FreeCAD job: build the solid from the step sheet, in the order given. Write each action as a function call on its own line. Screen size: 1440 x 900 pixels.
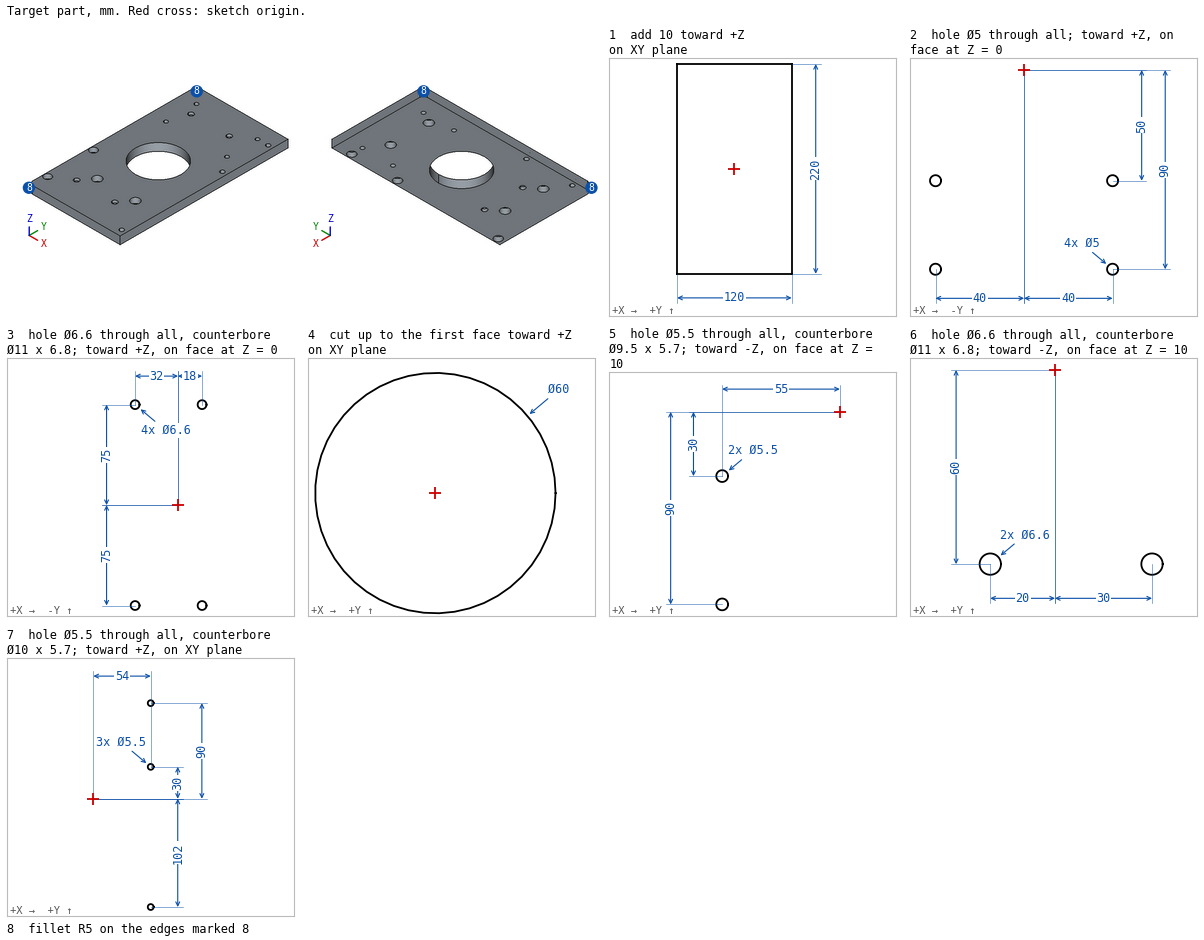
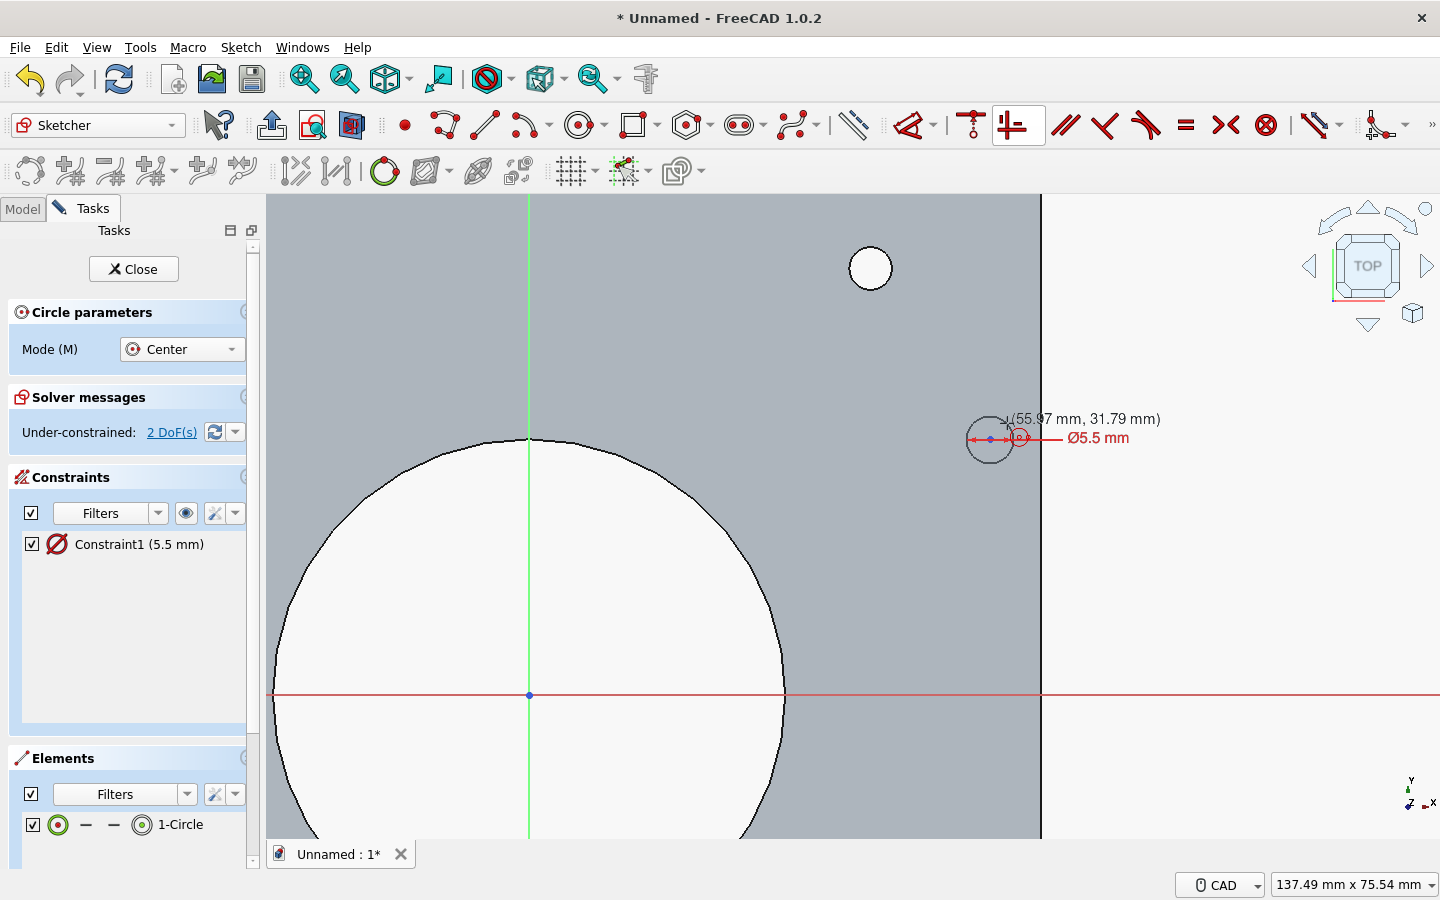
scroll(789, 441, down, 7)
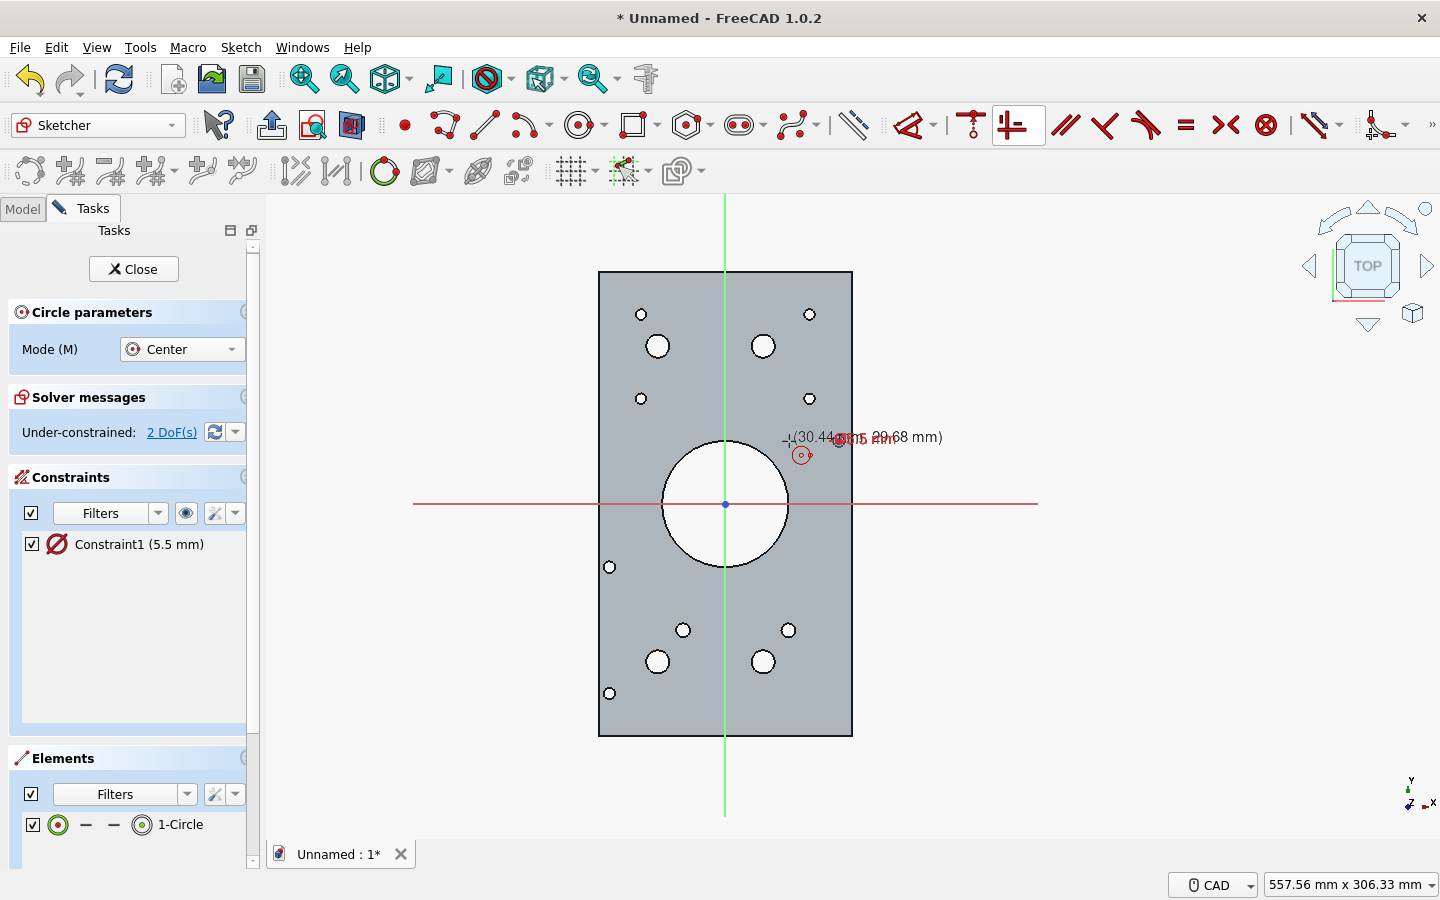
scroll(839, 315, up, 7)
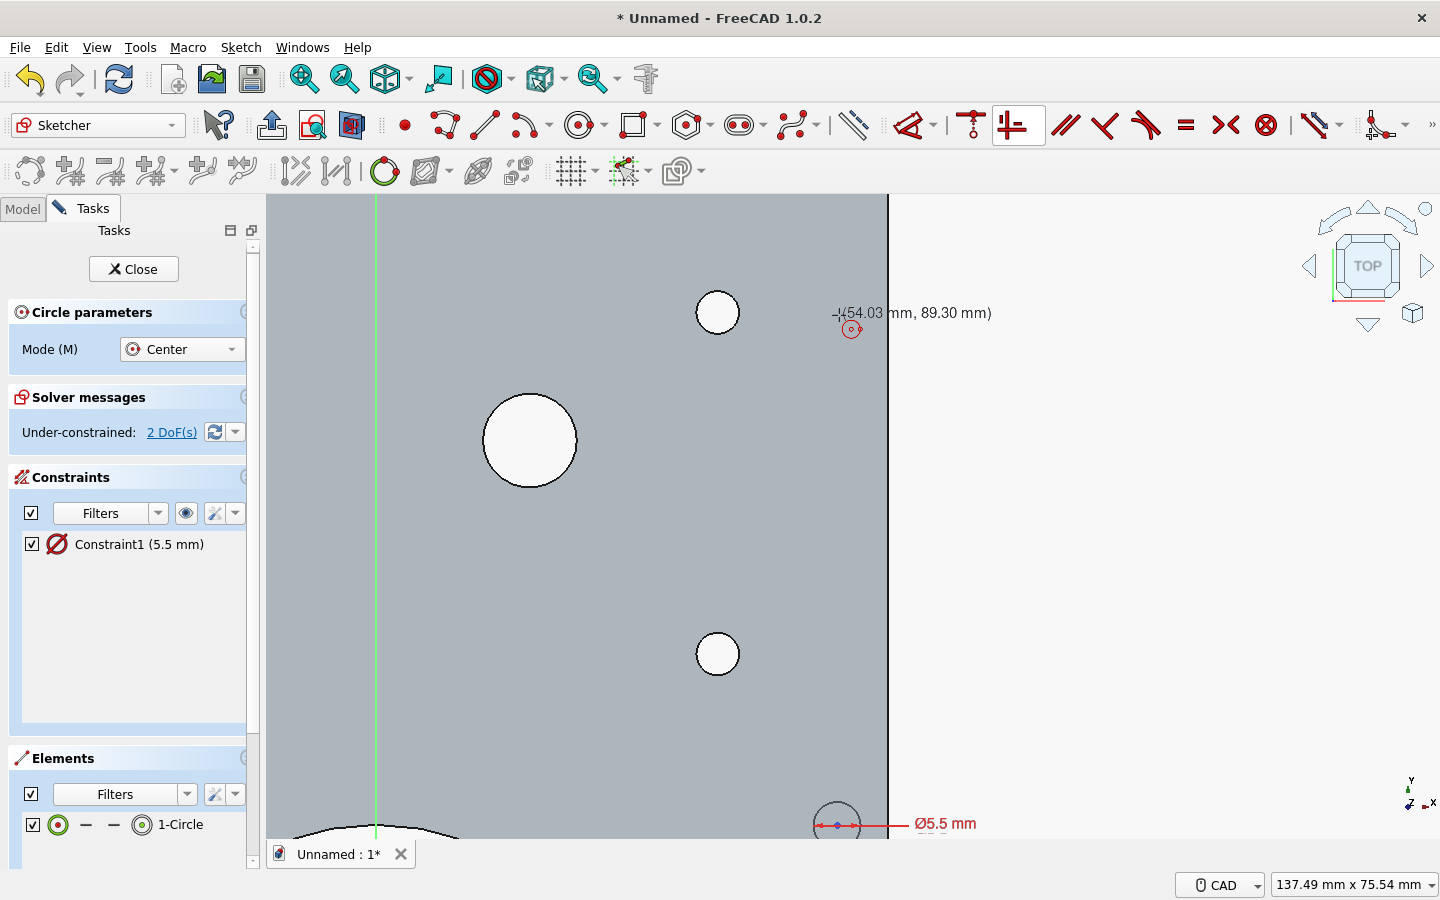
click(837, 313)
move(854, 296)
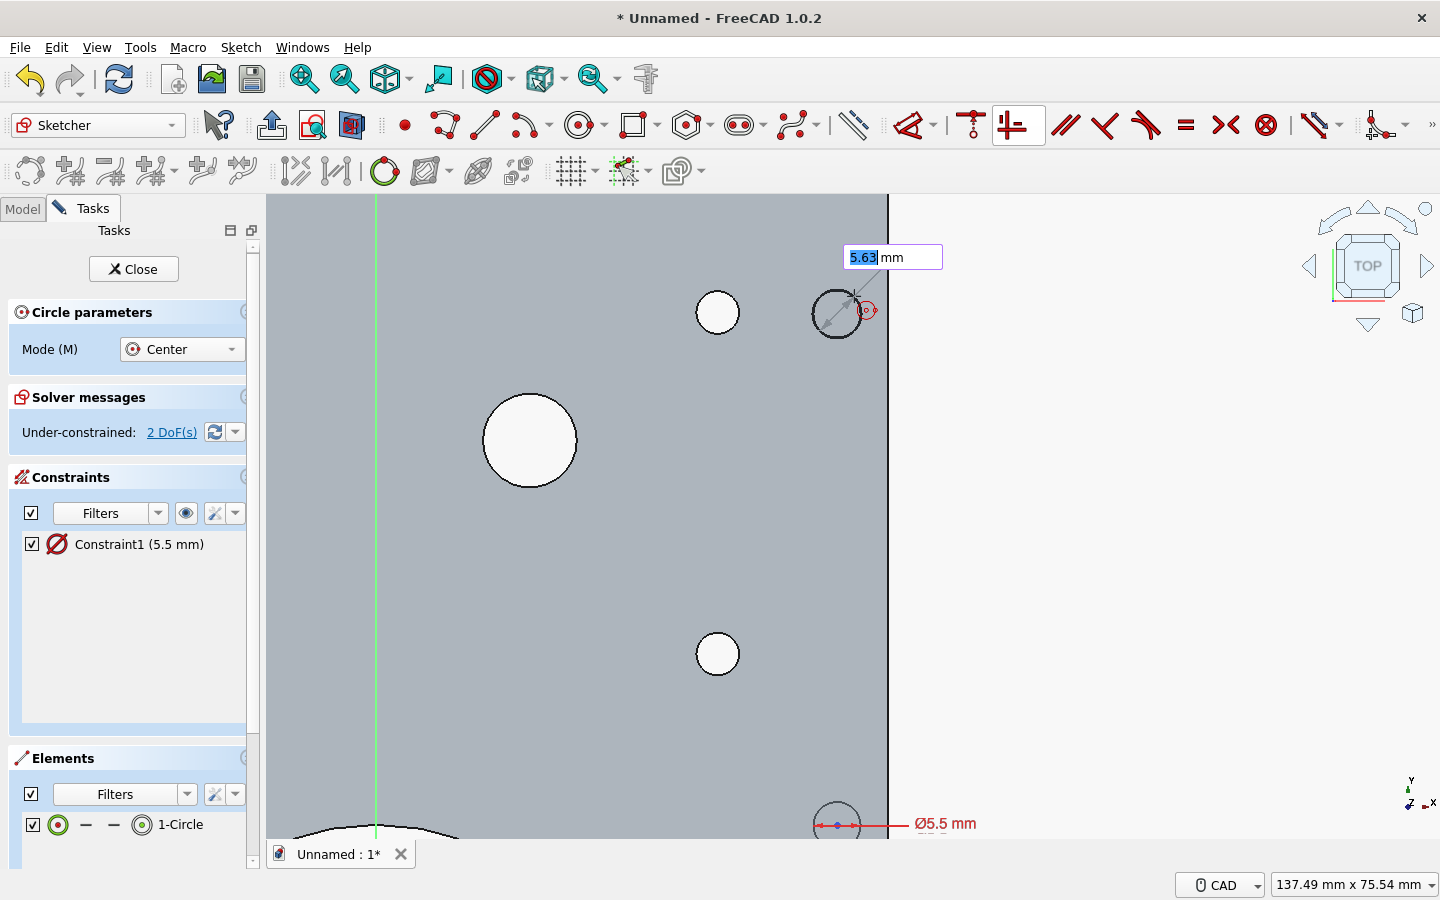
text(5.5)
key(Return)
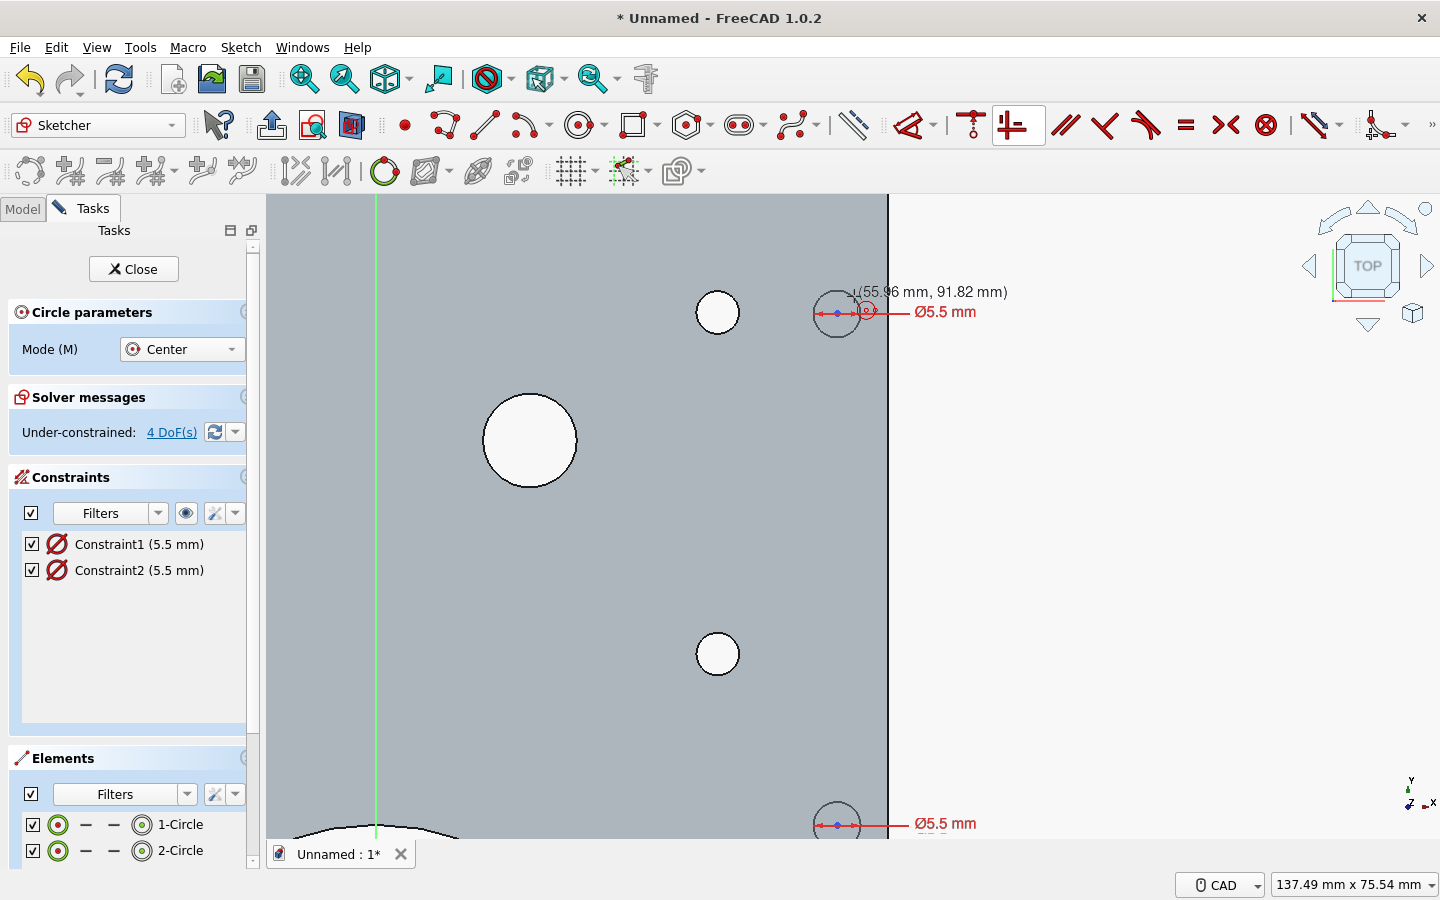
scroll(839, 315, down, 7)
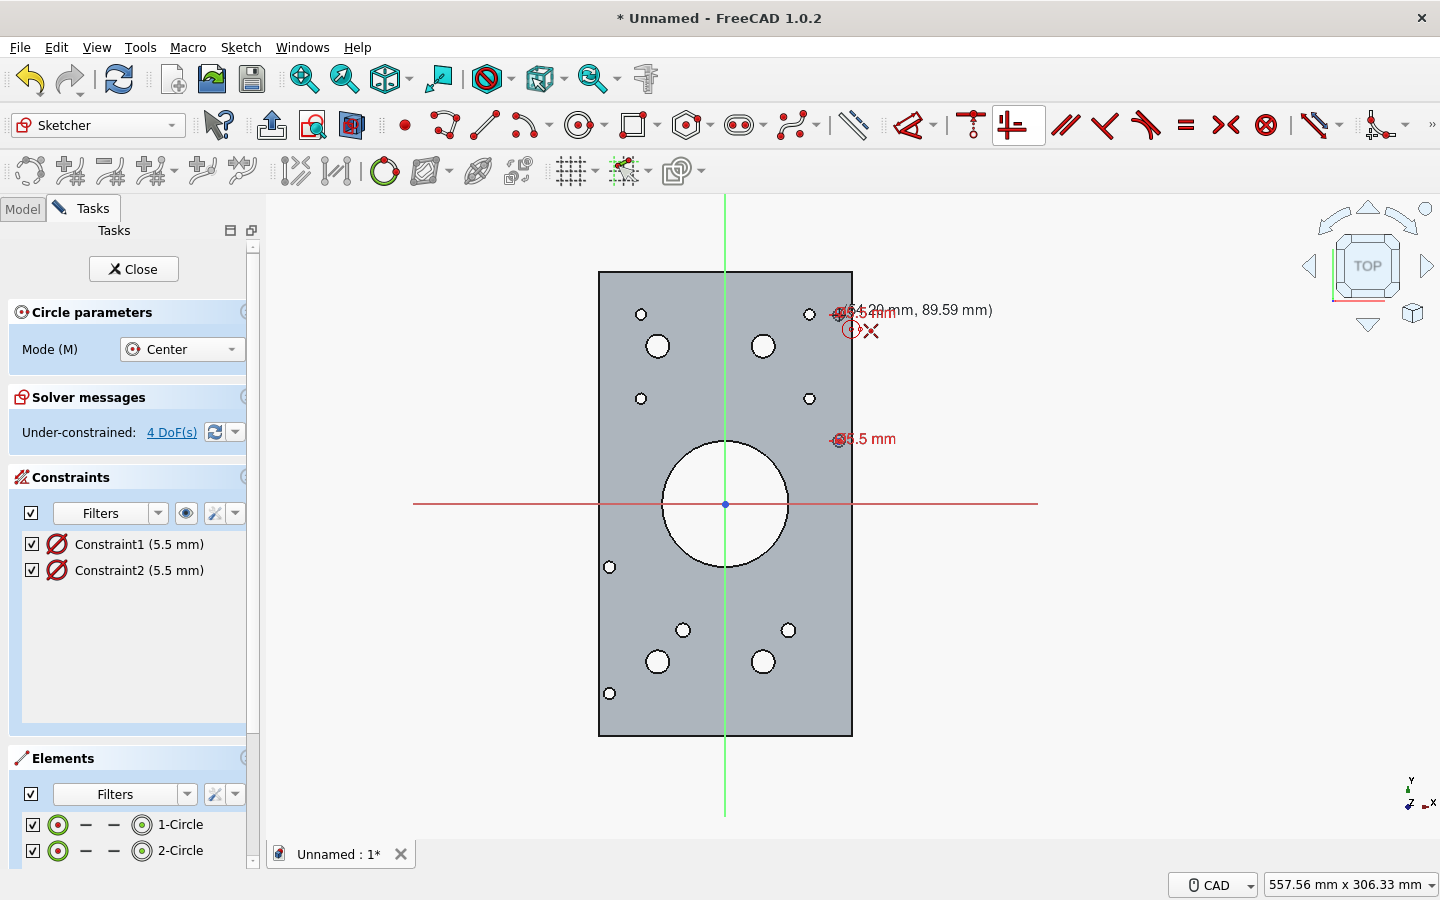
scroll(839, 719, up, 7)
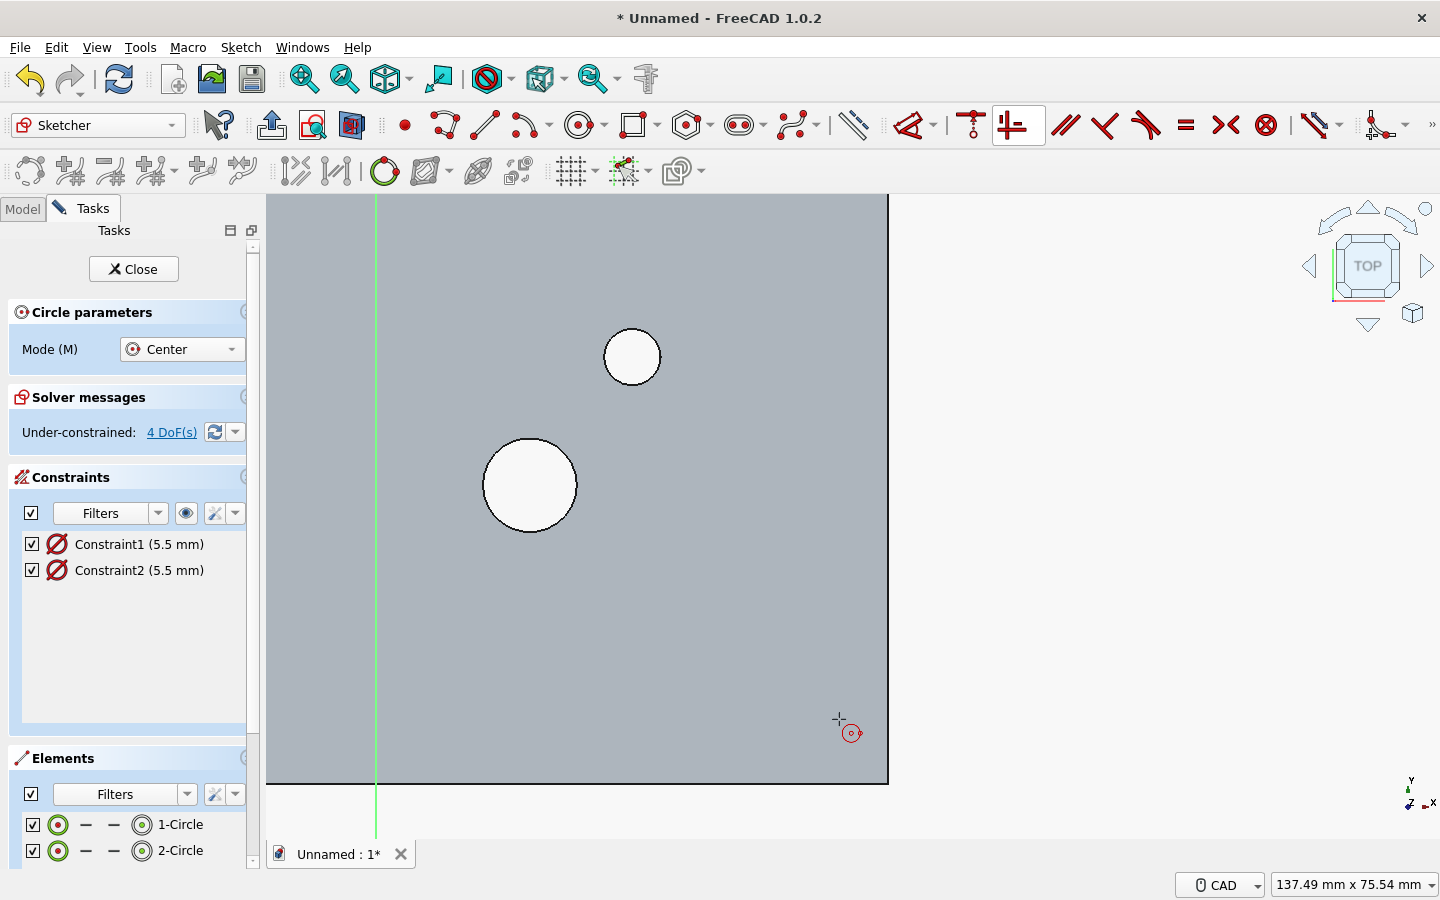
click(837, 716)
move(854, 699)